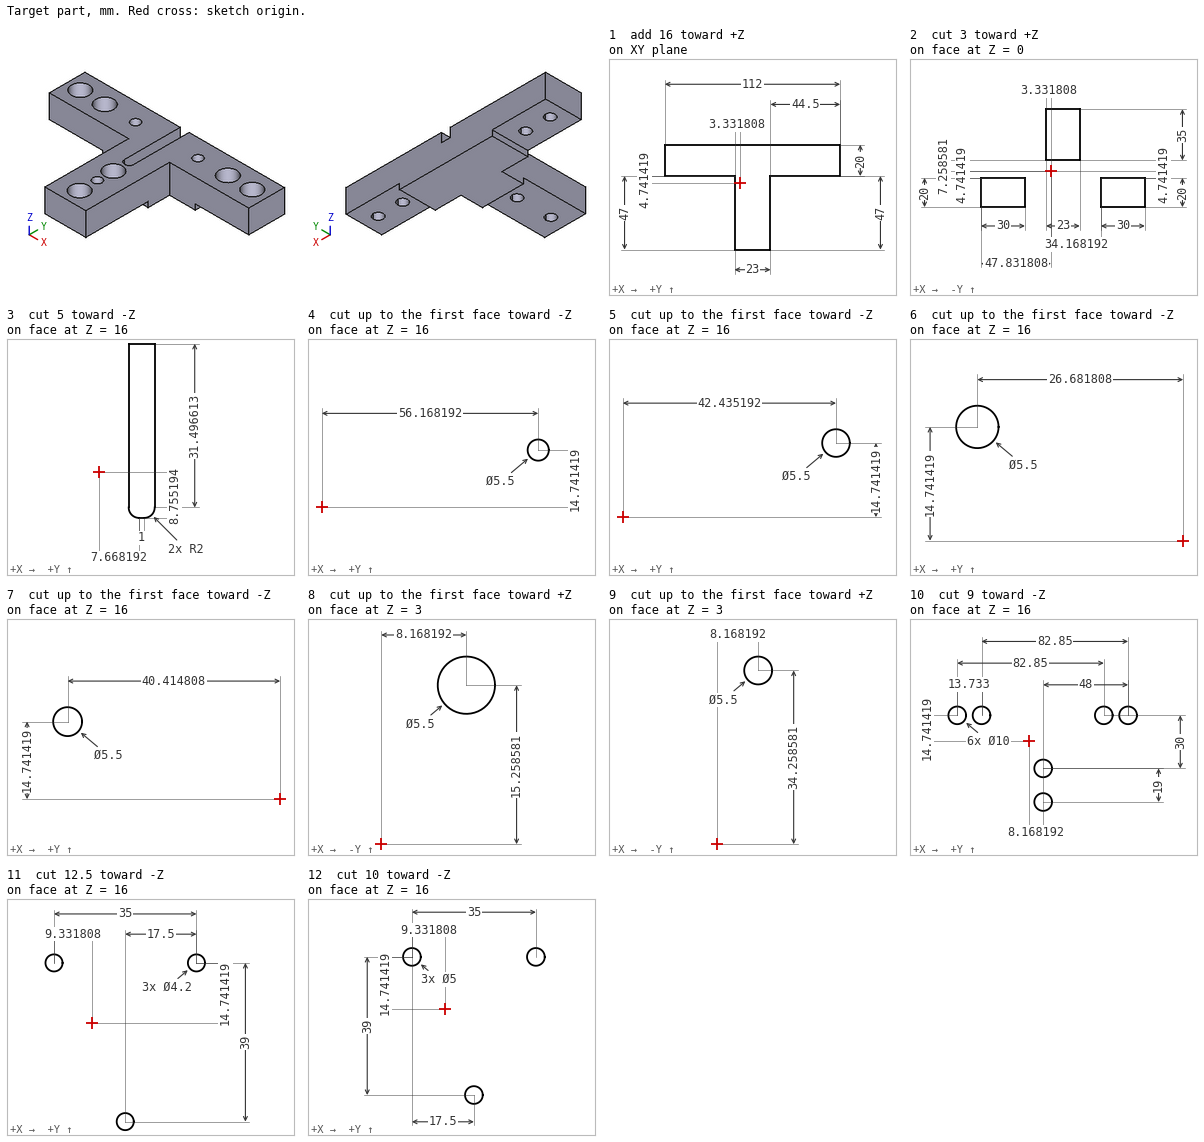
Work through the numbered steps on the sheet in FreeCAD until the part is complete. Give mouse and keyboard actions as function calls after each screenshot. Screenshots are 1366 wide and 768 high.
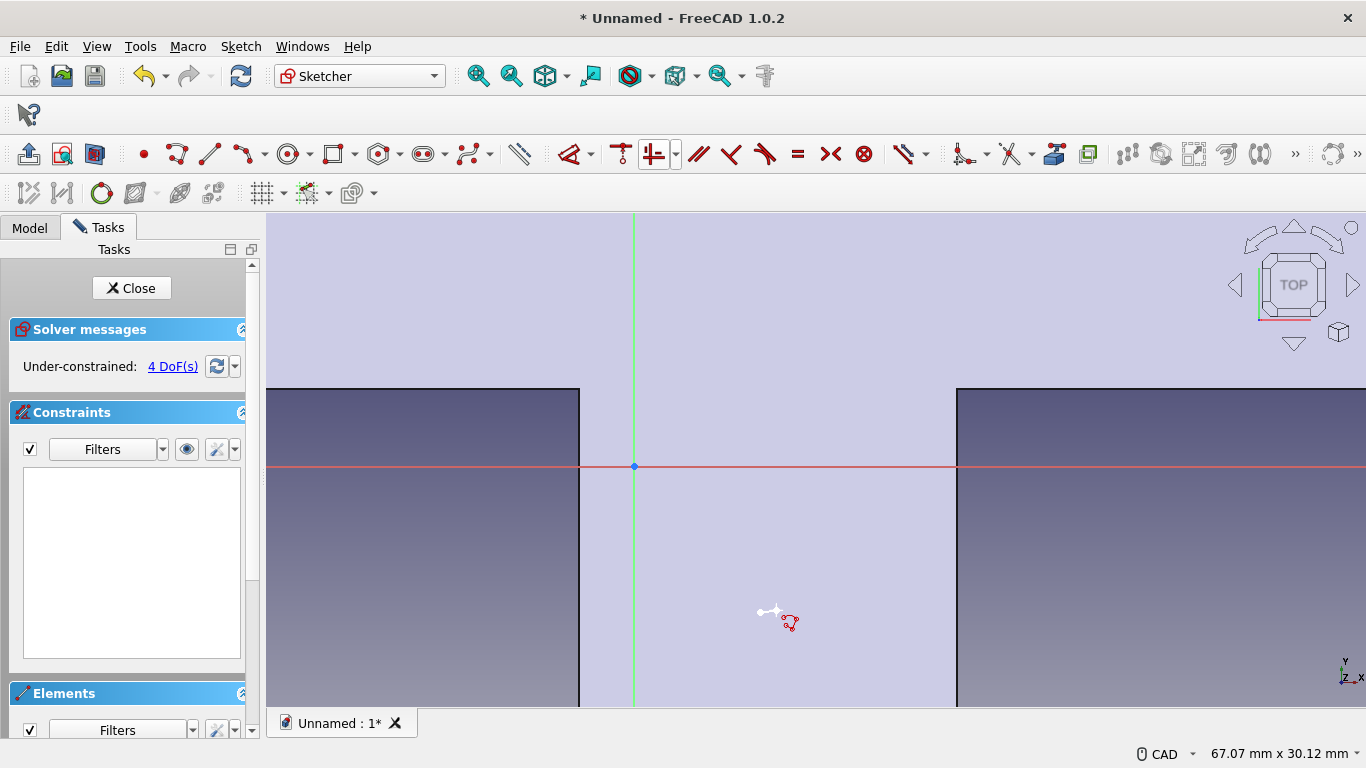
click(809, 577)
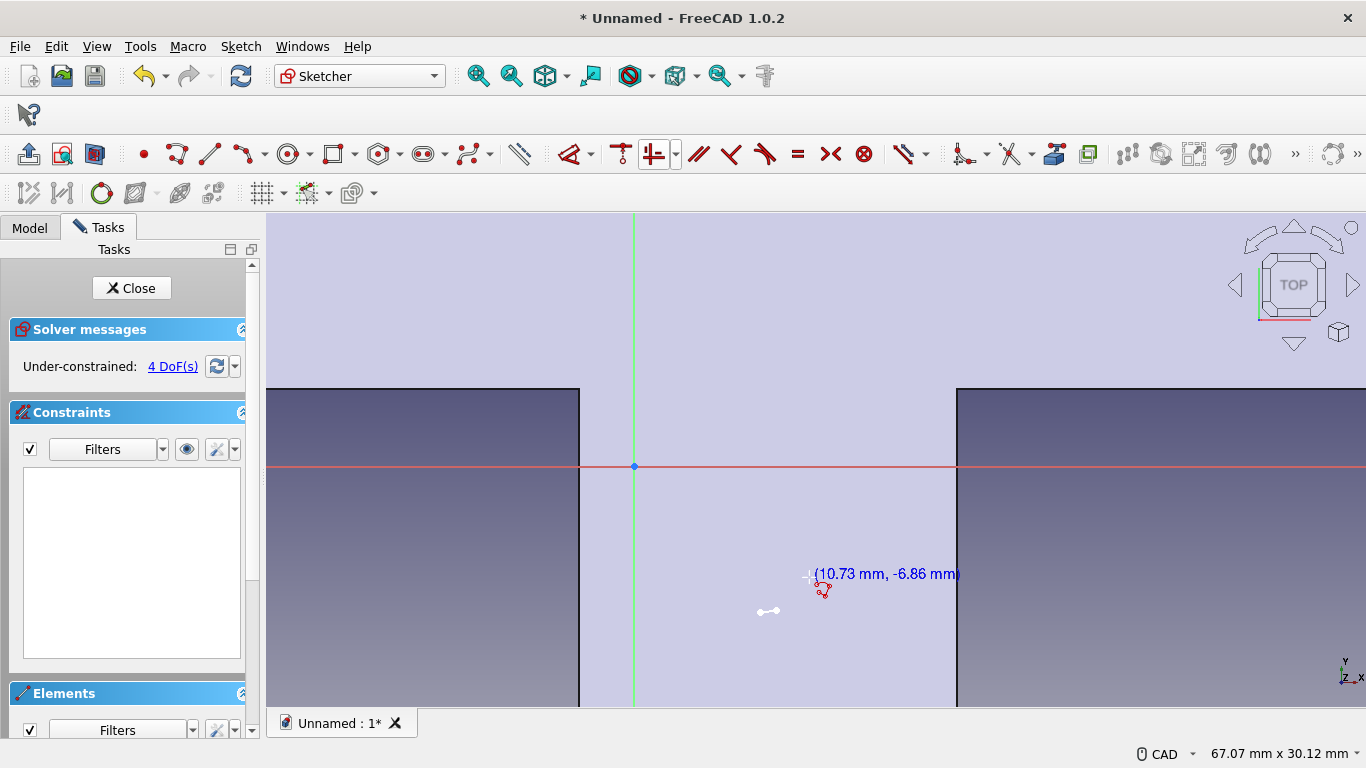
scroll(779, 612, down, 3)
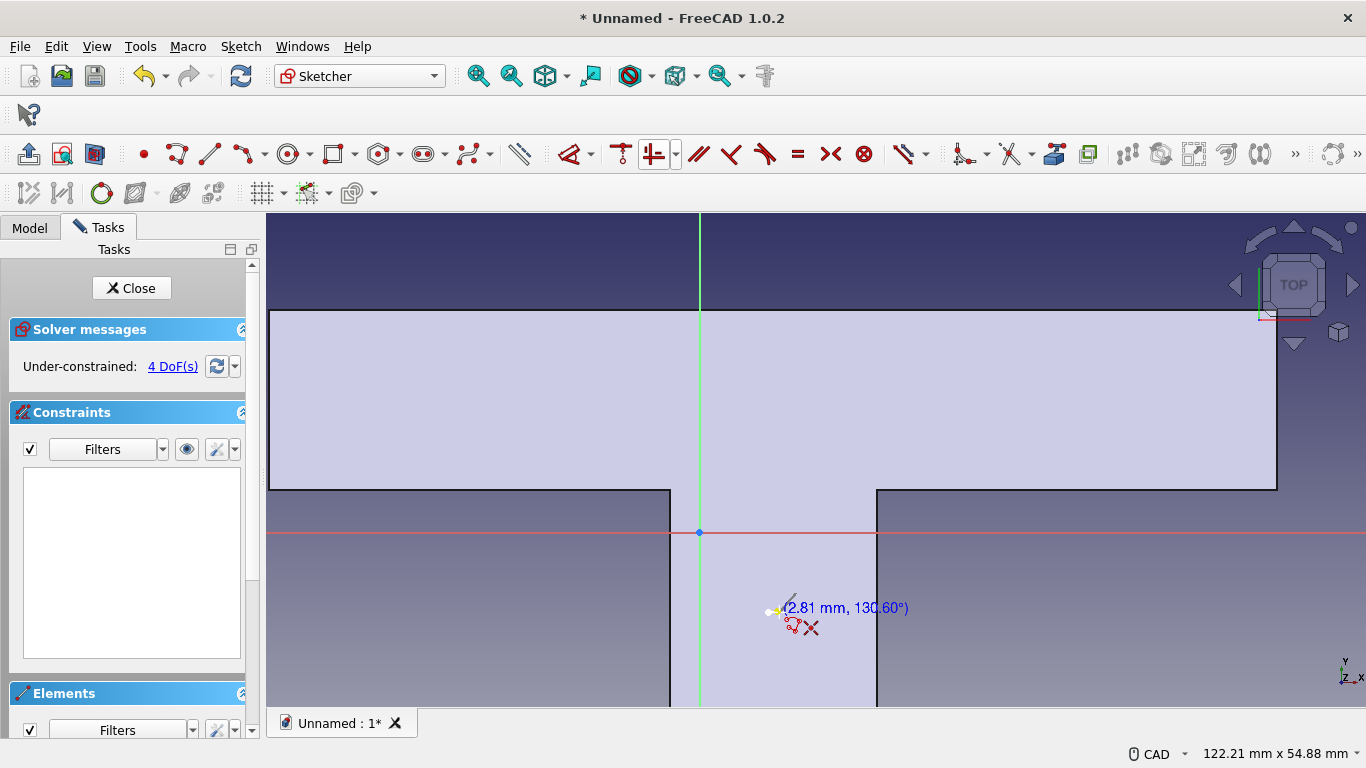
click(796, 310)
click(751, 310)
click(751, 593)
right_click(751, 593)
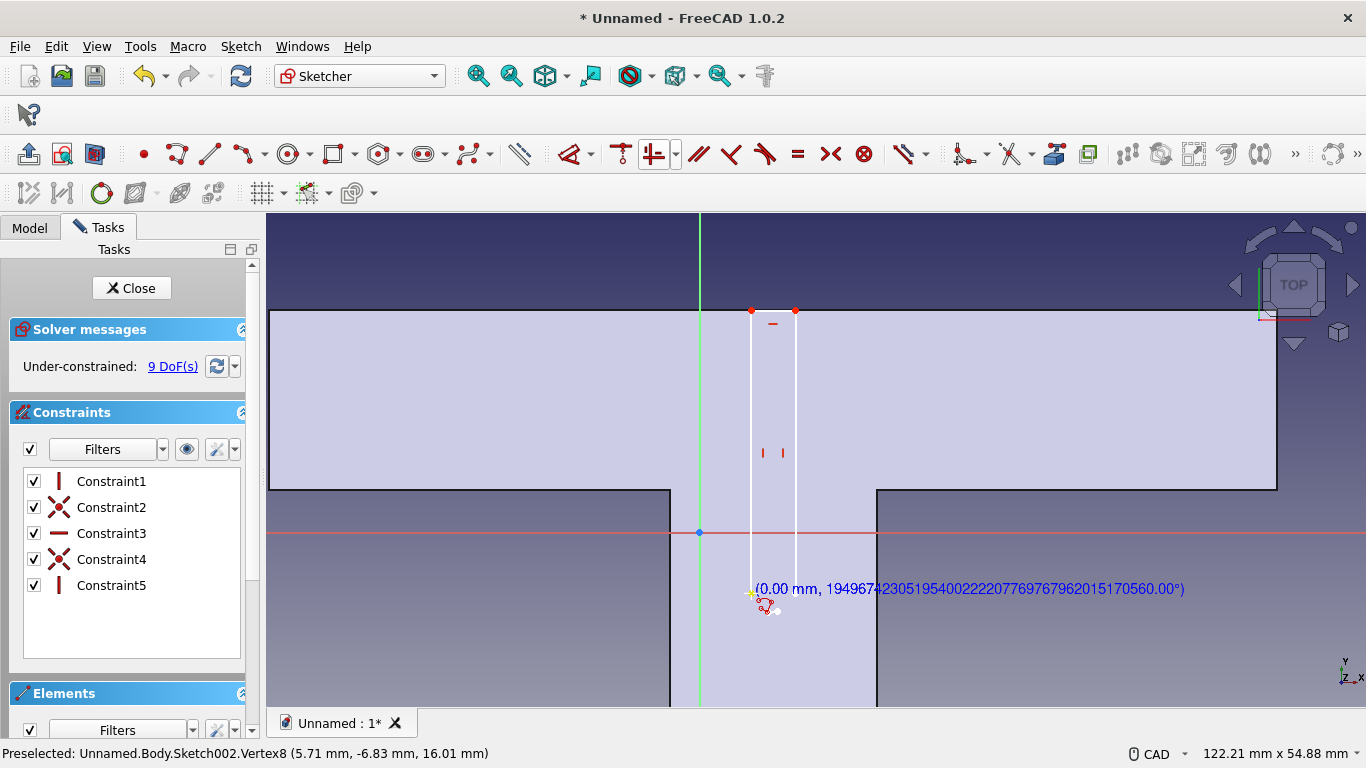
key(g)
key(3)
key(a)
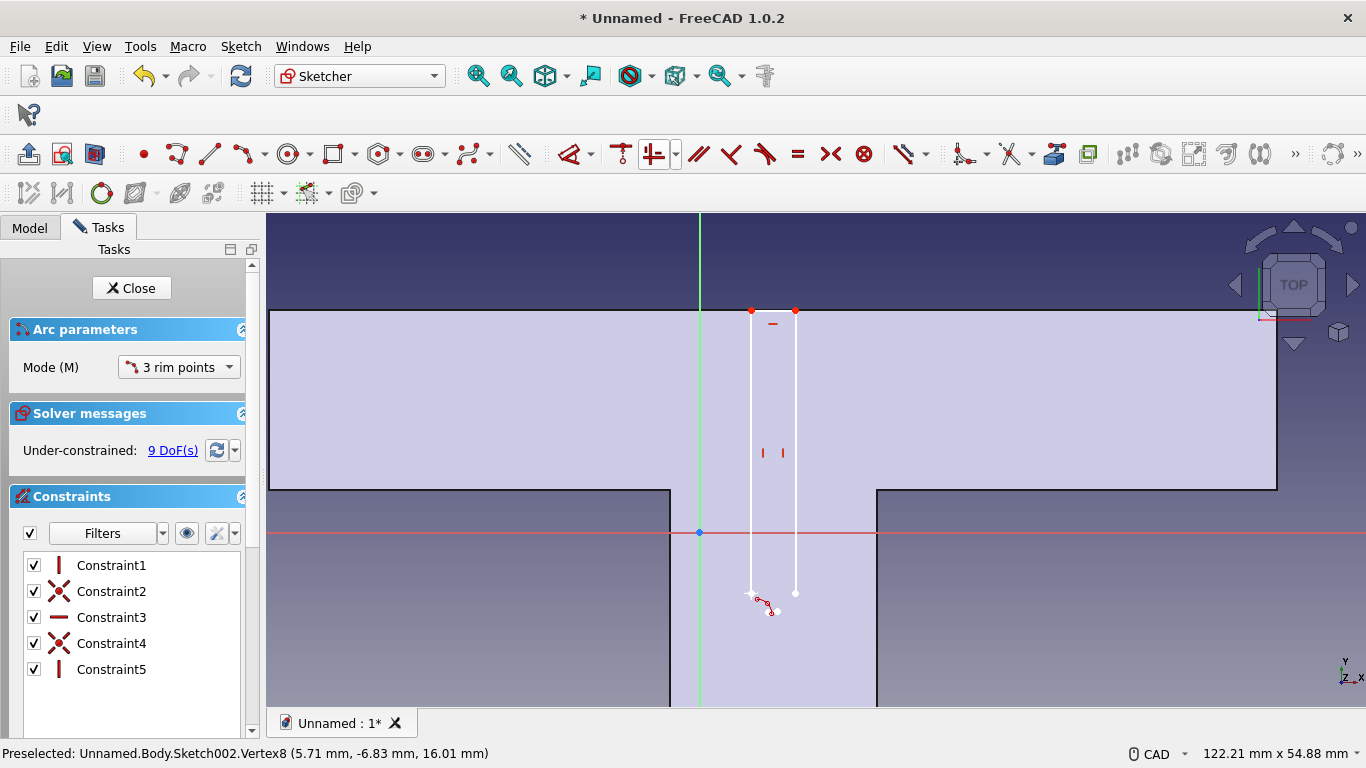
scroll(778, 611, up, 7)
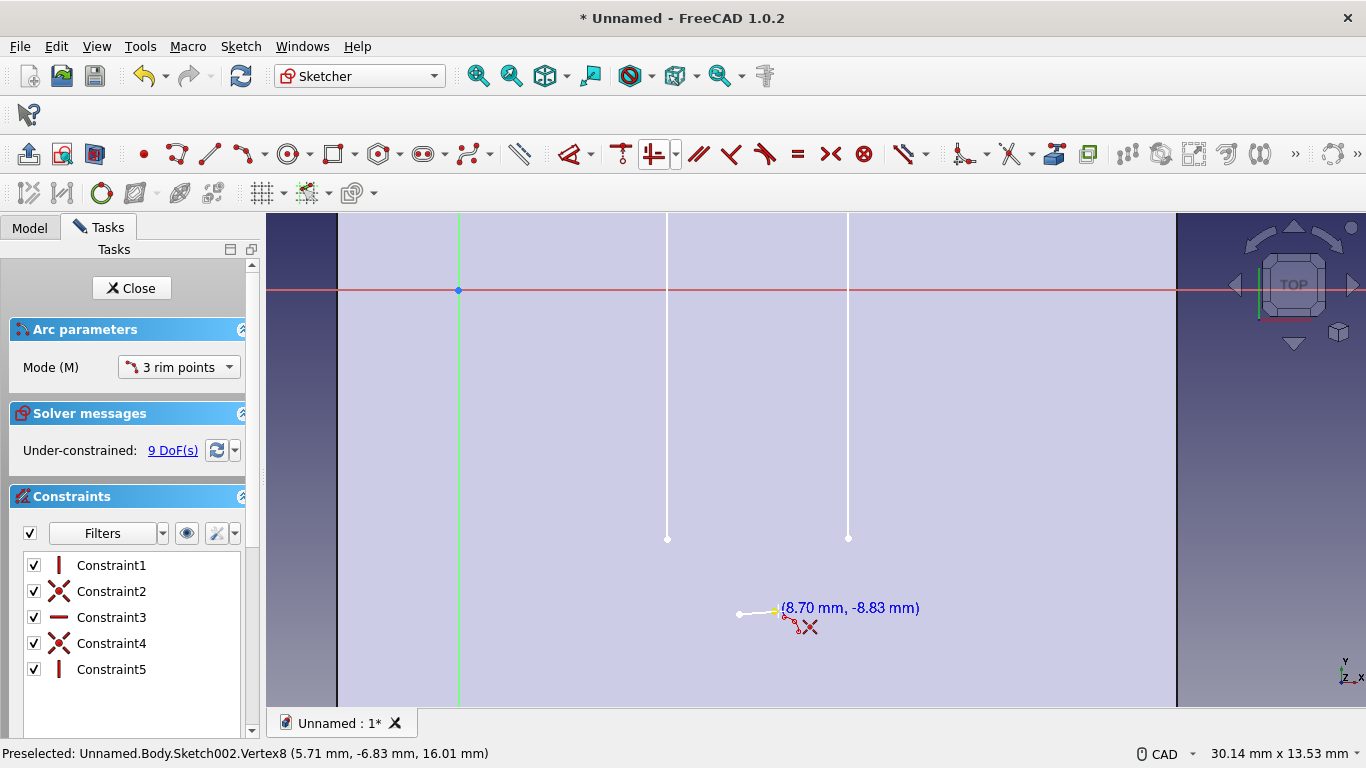
click(775, 612)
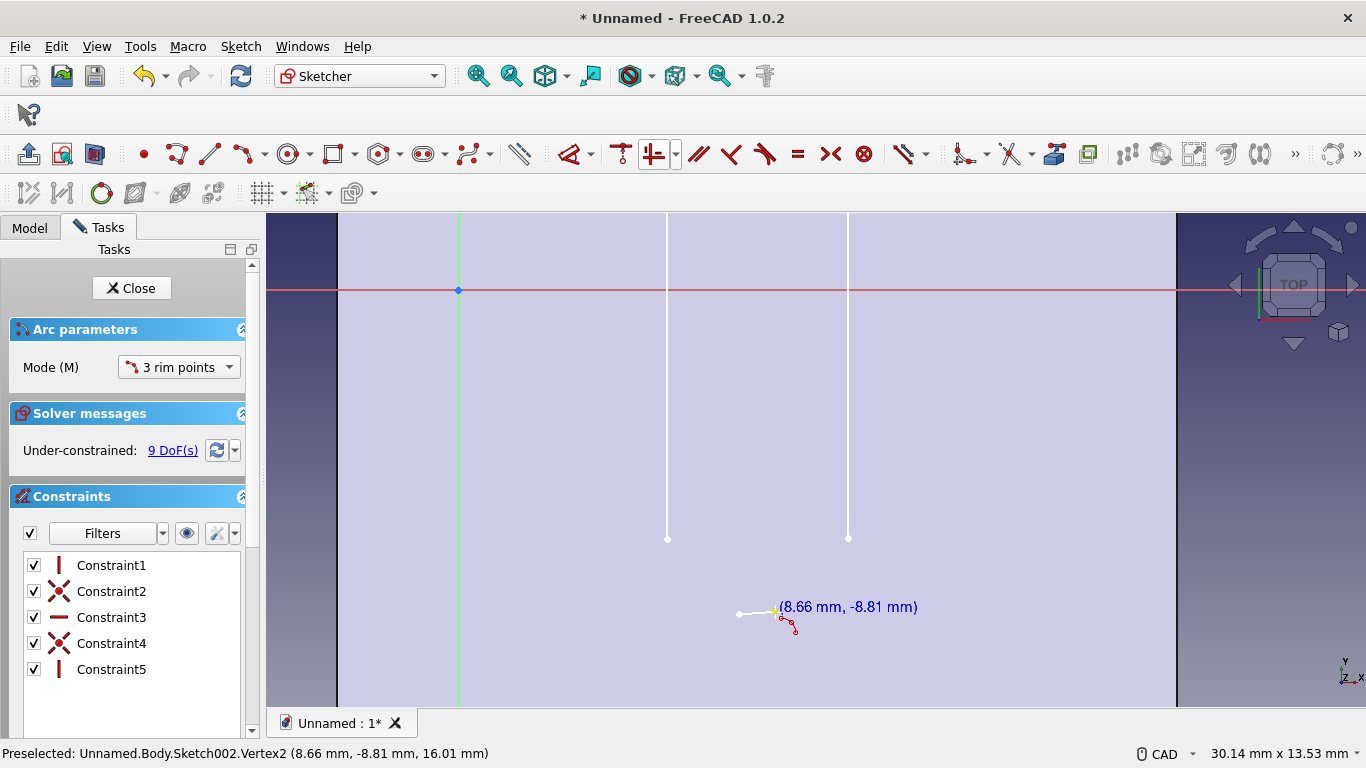
scroll(778, 611, down, 7)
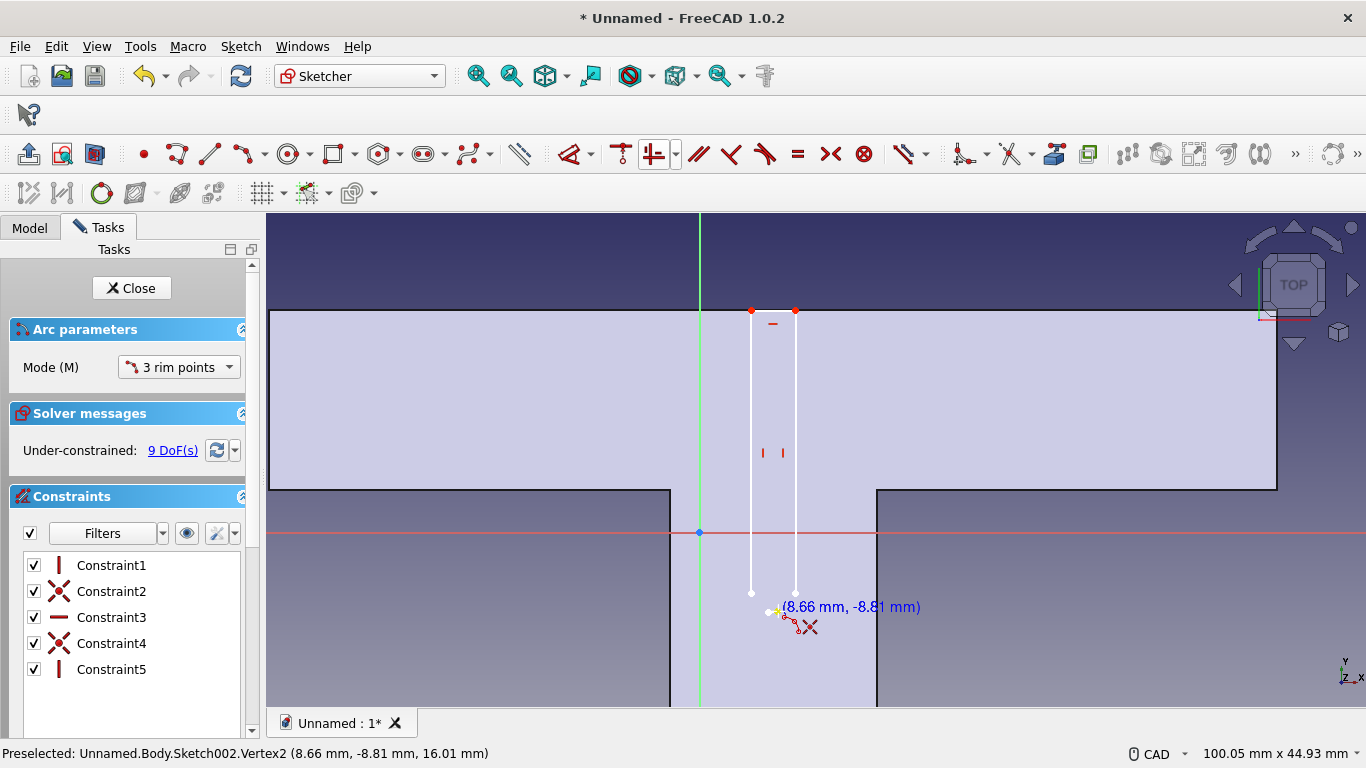
click(796, 594)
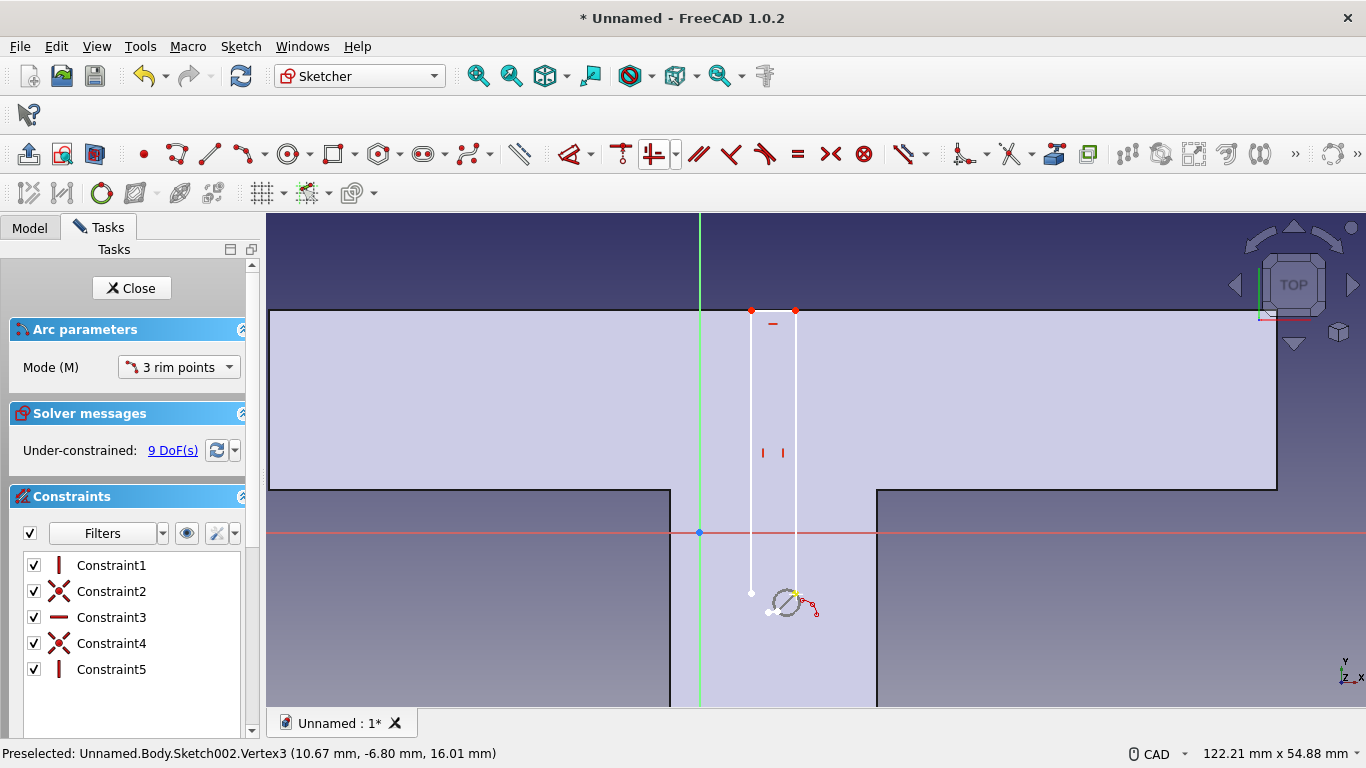
scroll(790, 606, up, 6)